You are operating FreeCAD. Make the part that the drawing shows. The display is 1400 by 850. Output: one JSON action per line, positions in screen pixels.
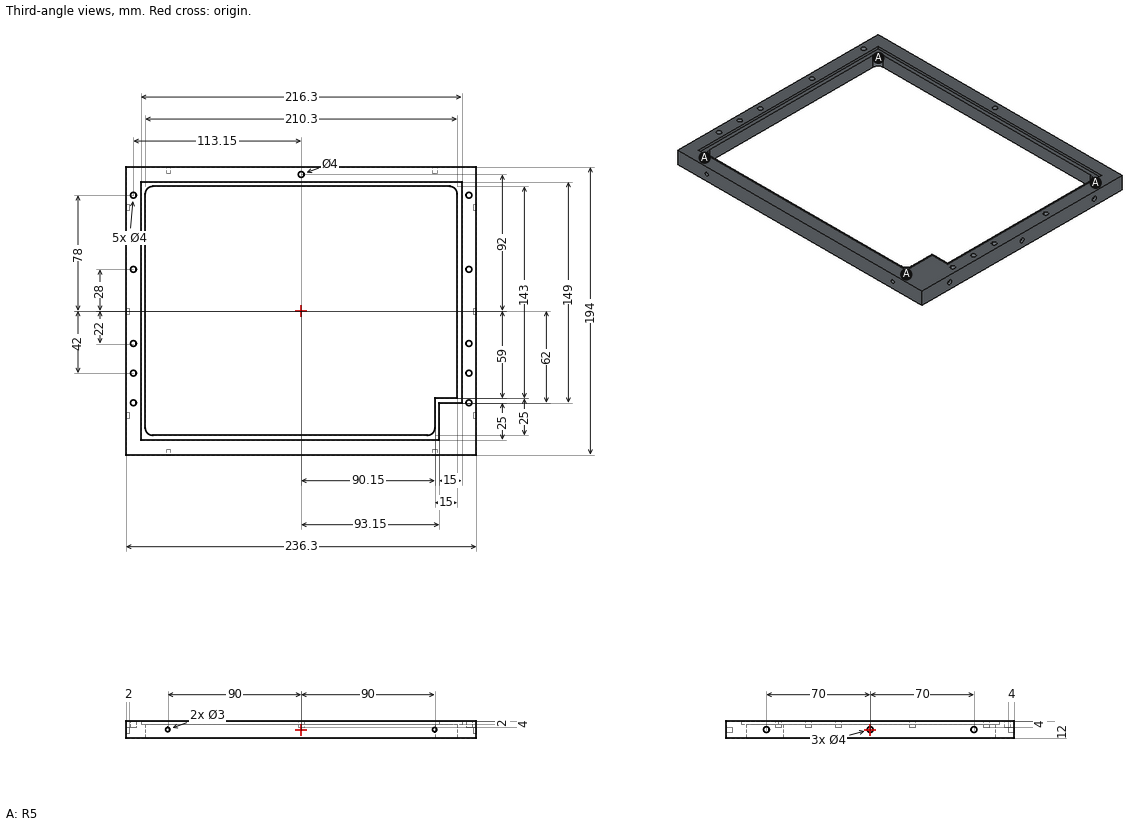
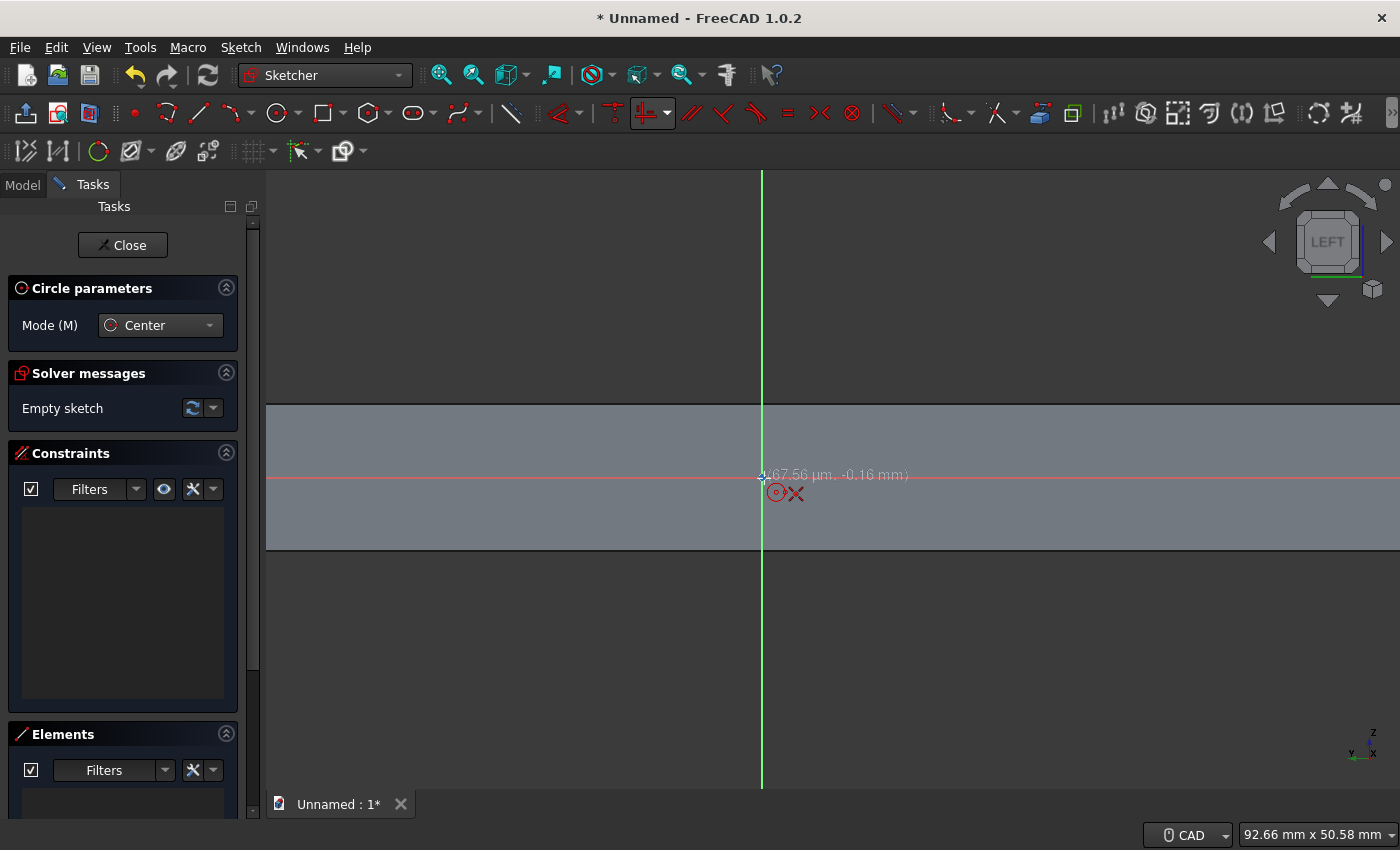
{"action": "left_click", "coordinate": [762, 478]}
{"action": "left_click", "coordinate": [780, 461]}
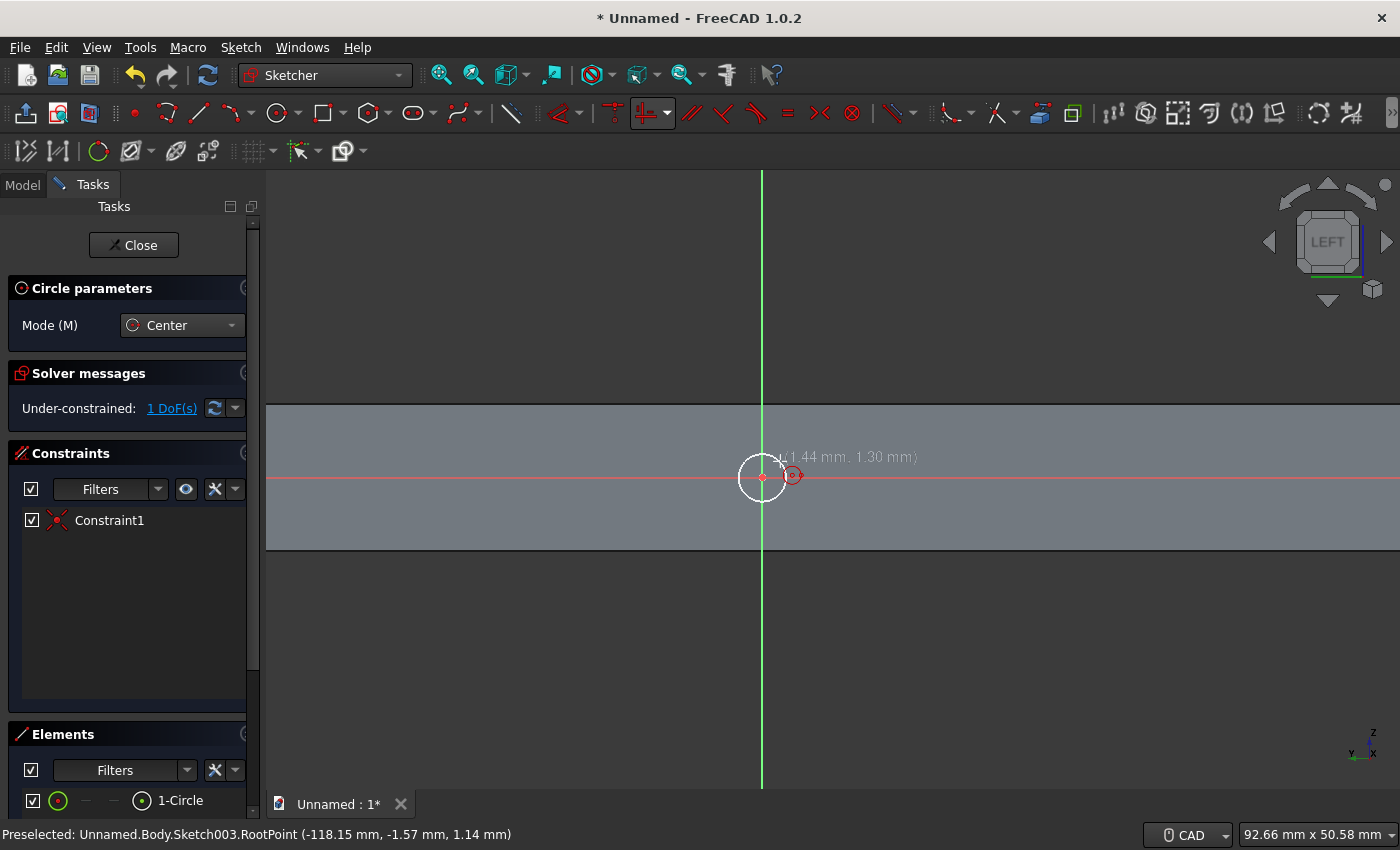
{"action": "scroll", "coordinate": [766, 480], "scroll_direction": "down", "scroll_amount": 5}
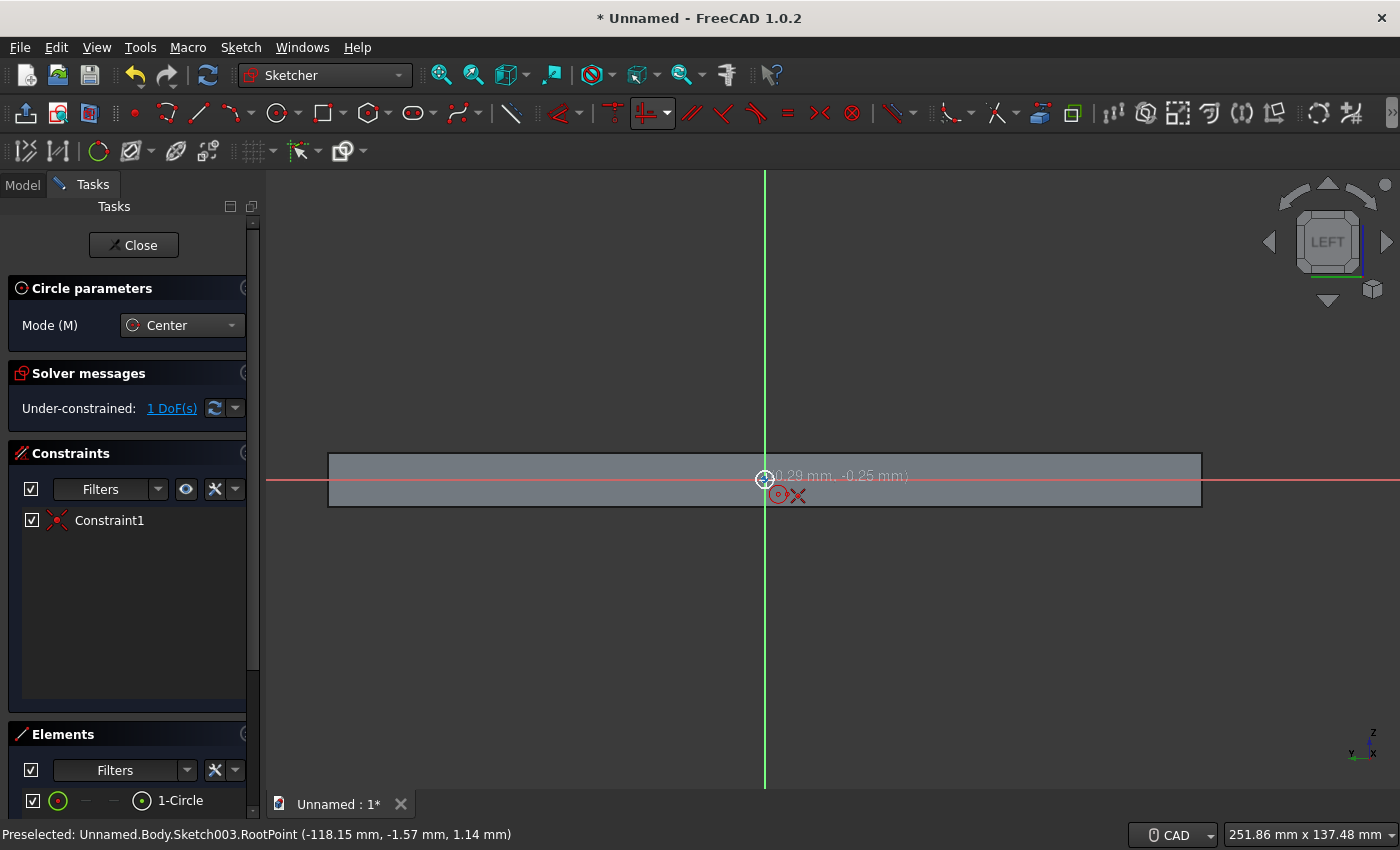
{"action": "scroll", "coordinate": [450, 480], "scroll_direction": "up", "scroll_amount": 5}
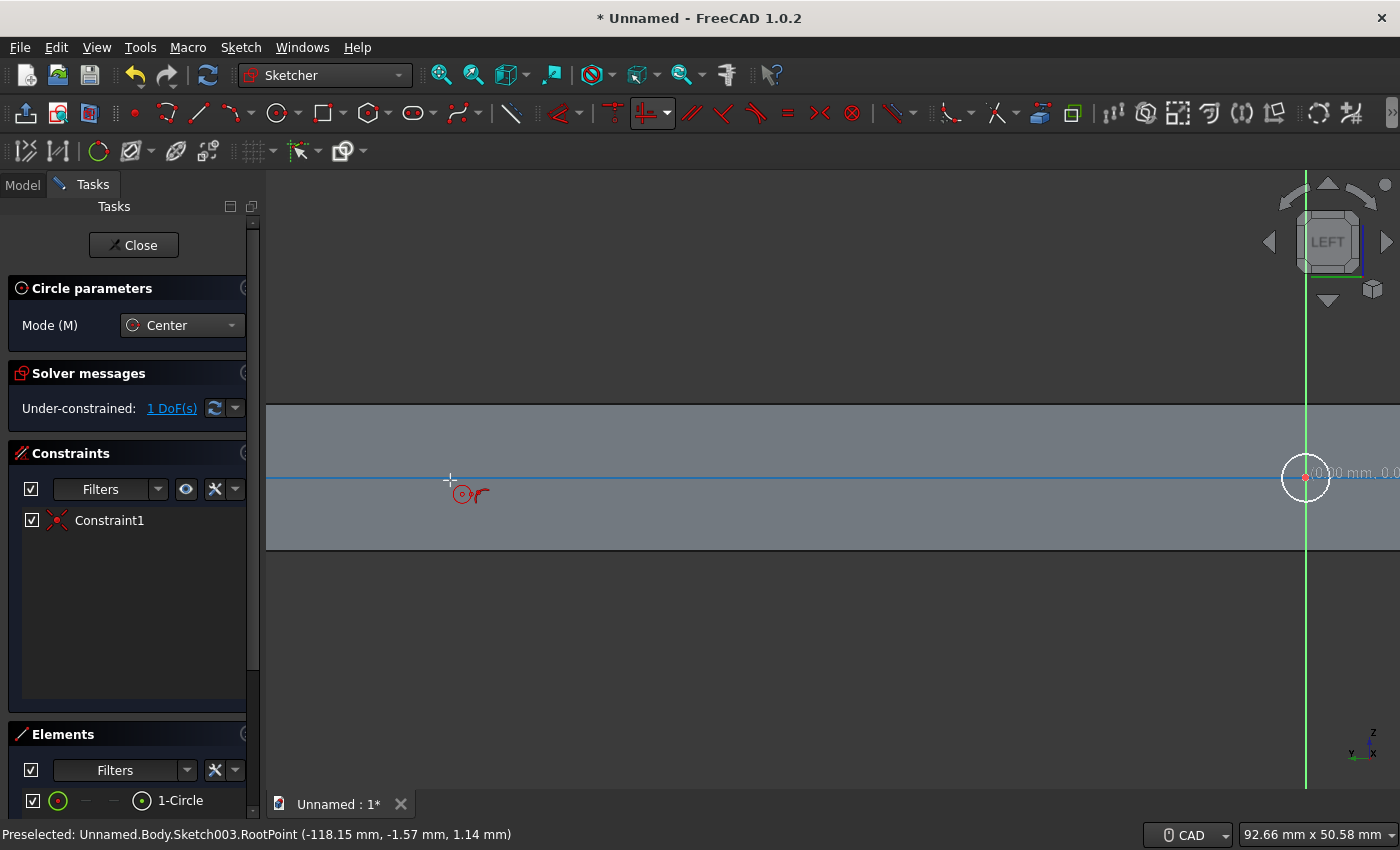
{"action": "left_click", "coordinate": [449, 478]}
{"action": "left_click", "coordinate": [466, 461]}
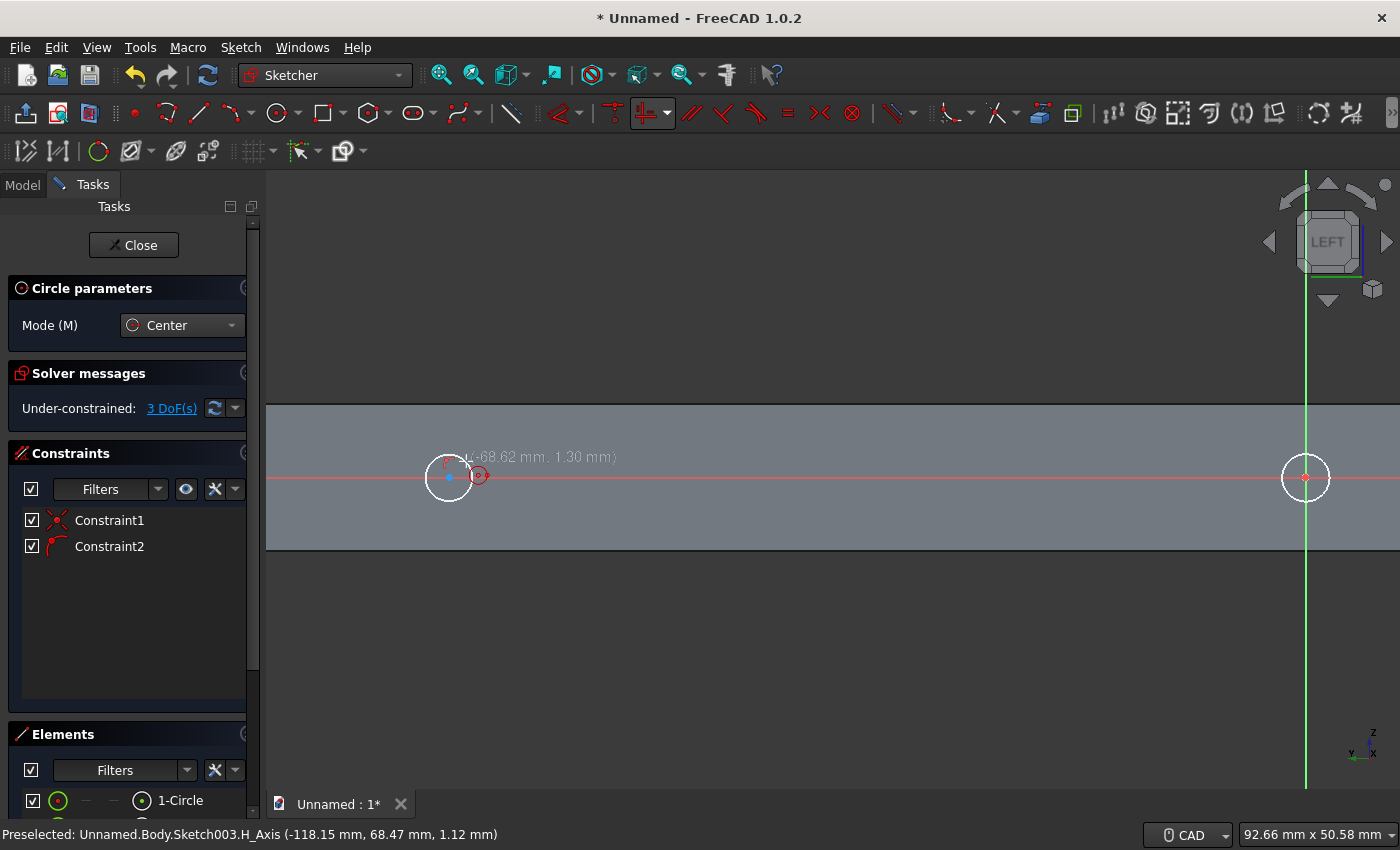
{"action": "scroll", "coordinate": [449, 480], "scroll_direction": "down", "scroll_amount": 5}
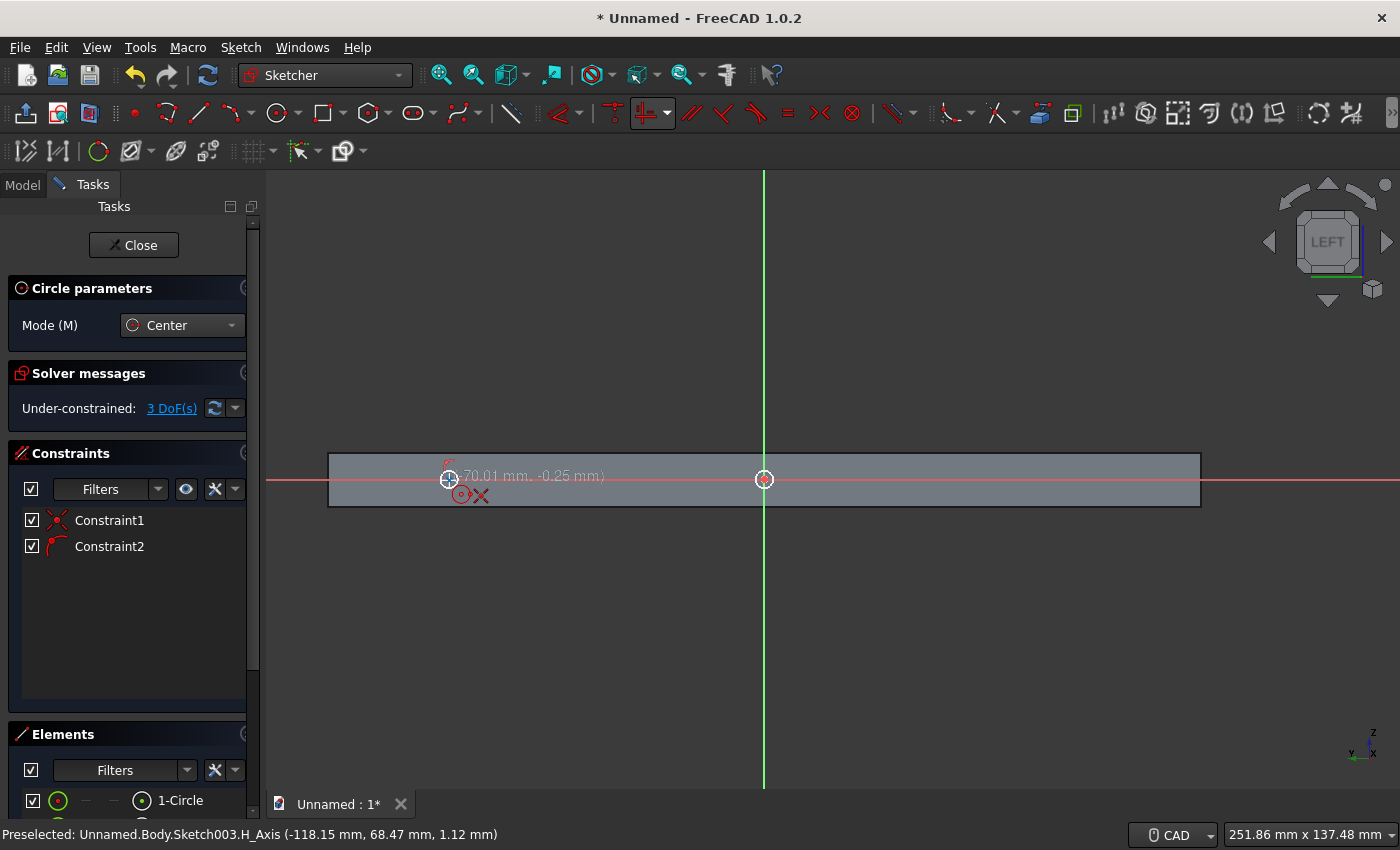
{"action": "scroll", "coordinate": [1079, 480], "scroll_direction": "up", "scroll_amount": 5}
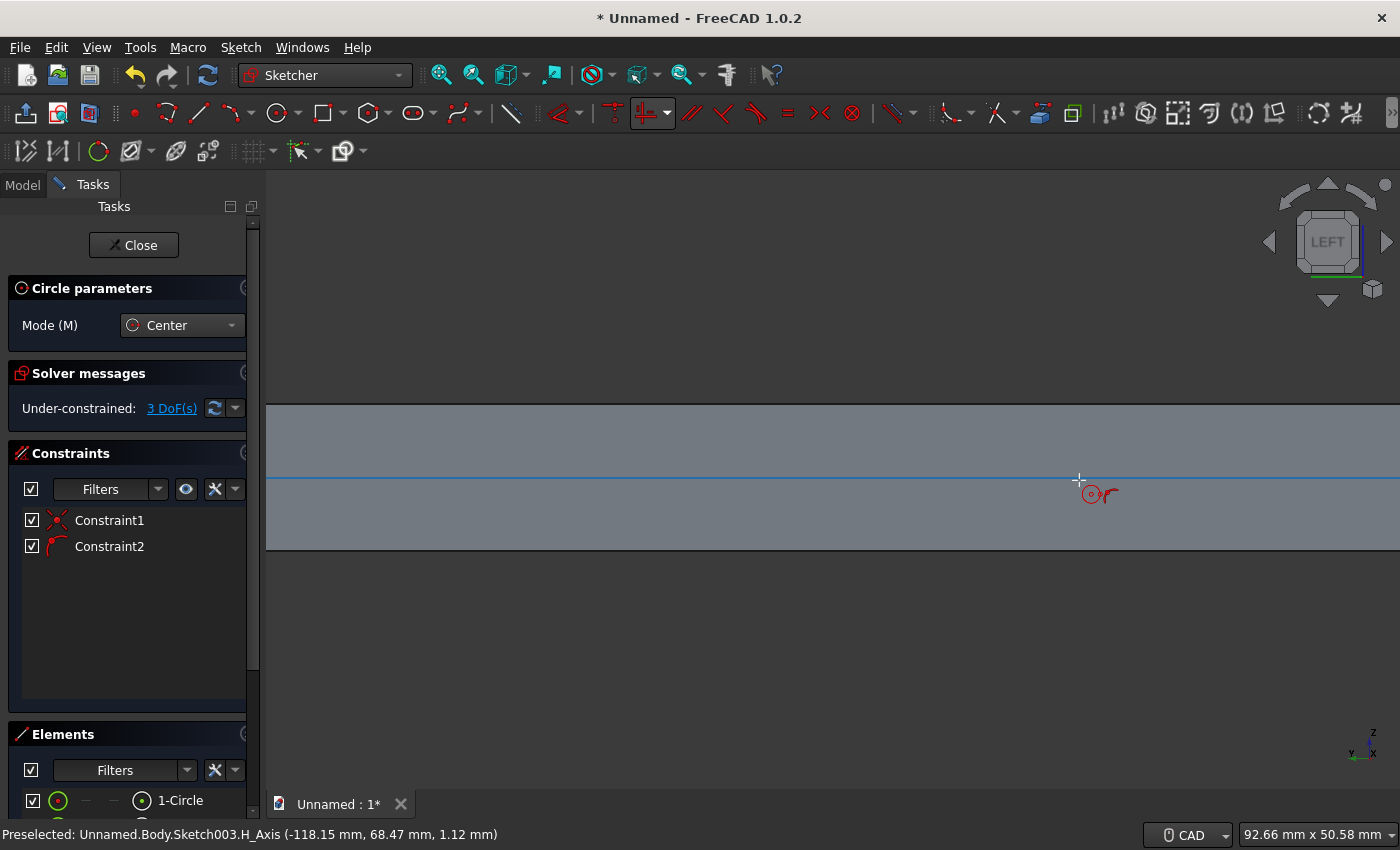
{"action": "left_click", "coordinate": [1079, 478]}
{"action": "left_click", "coordinate": [1096, 461]}
{"action": "key", "text": "Escape"}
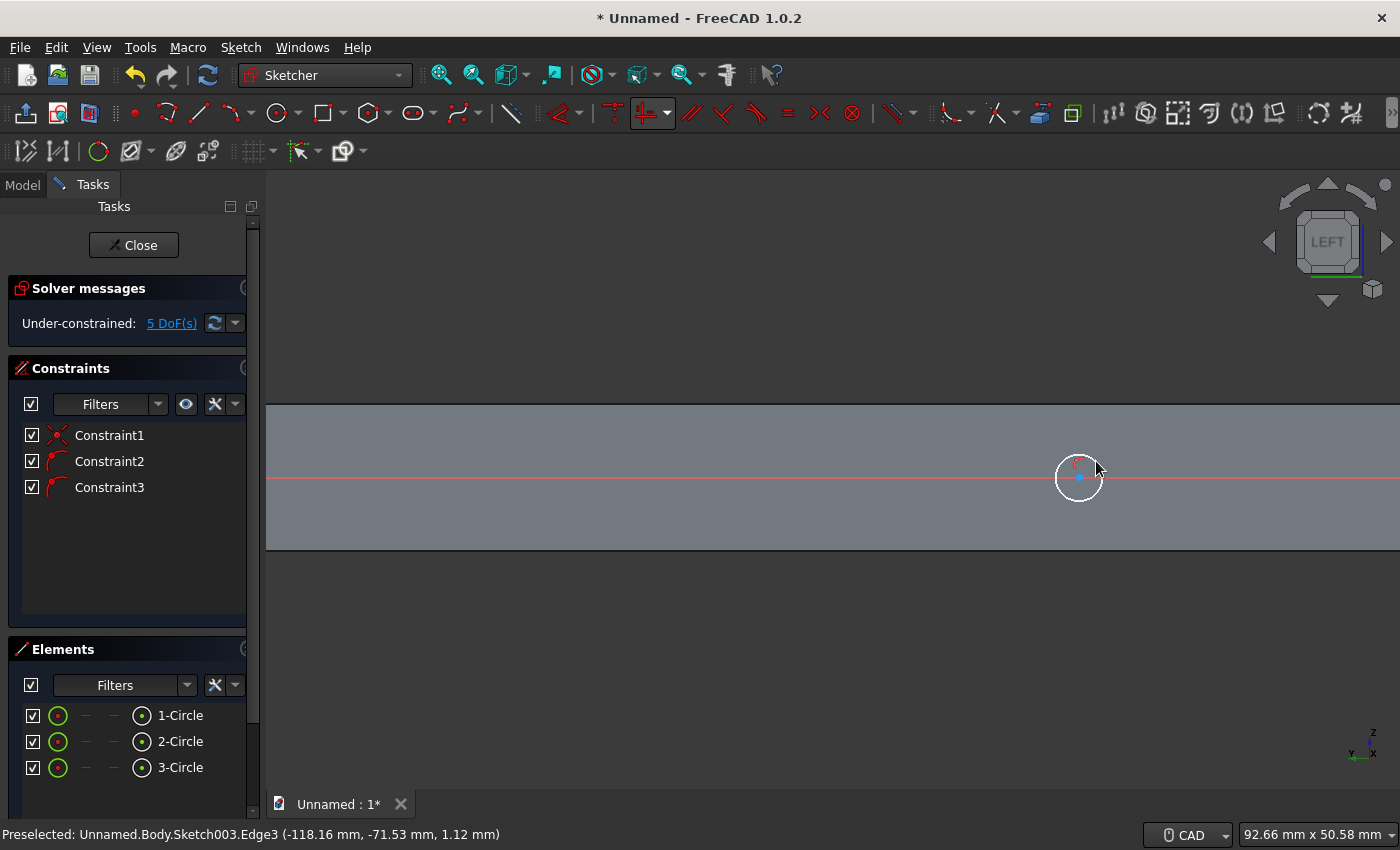
{"action": "scroll", "coordinate": [1080, 480], "scroll_direction": "down", "scroll_amount": 5}